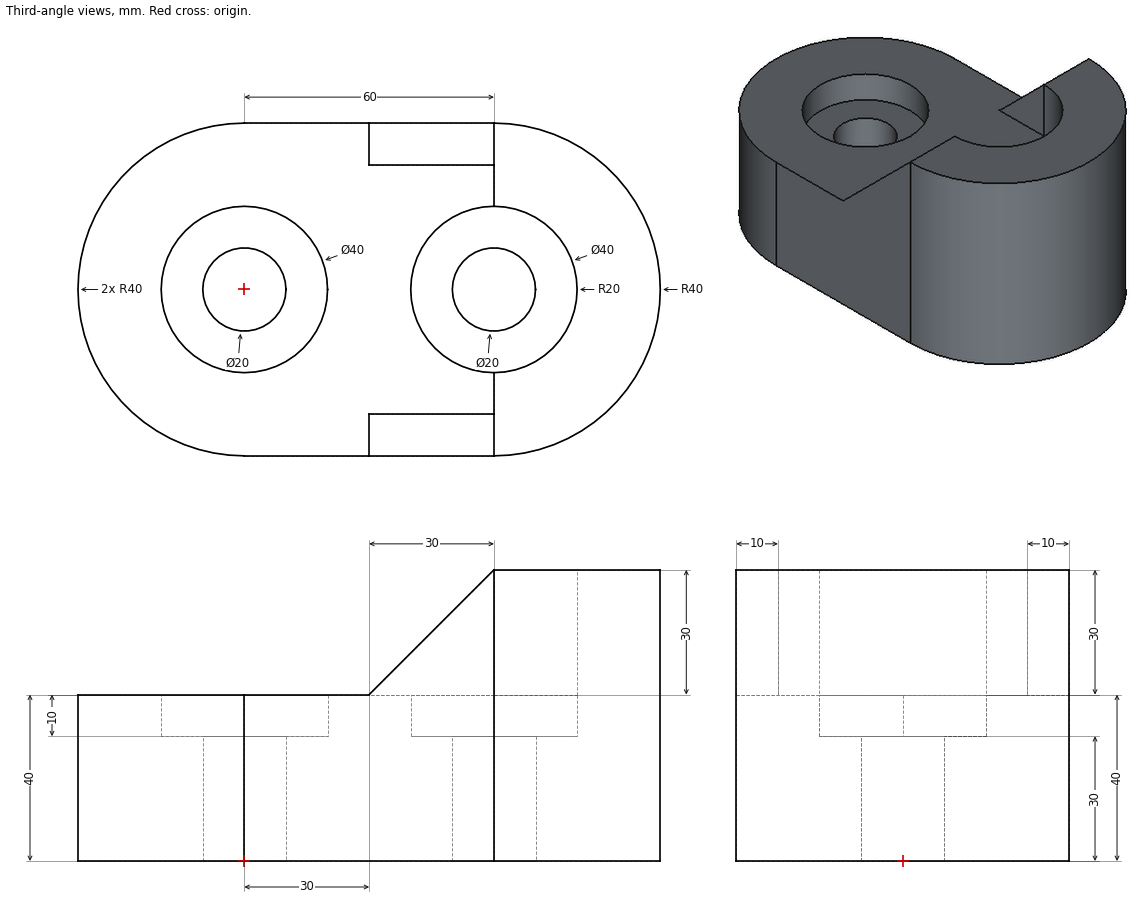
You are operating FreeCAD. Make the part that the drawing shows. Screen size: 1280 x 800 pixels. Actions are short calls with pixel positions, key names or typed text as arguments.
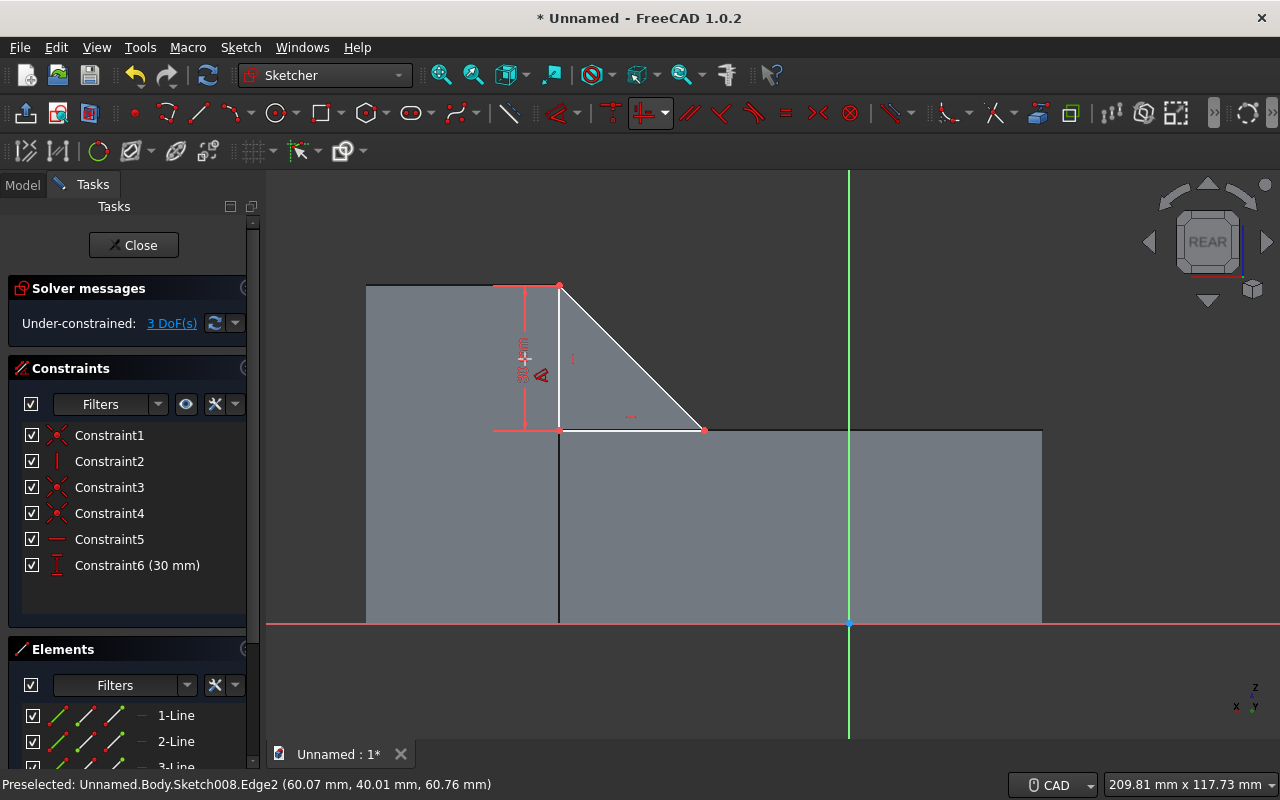
click(603, 431)
click(631, 397)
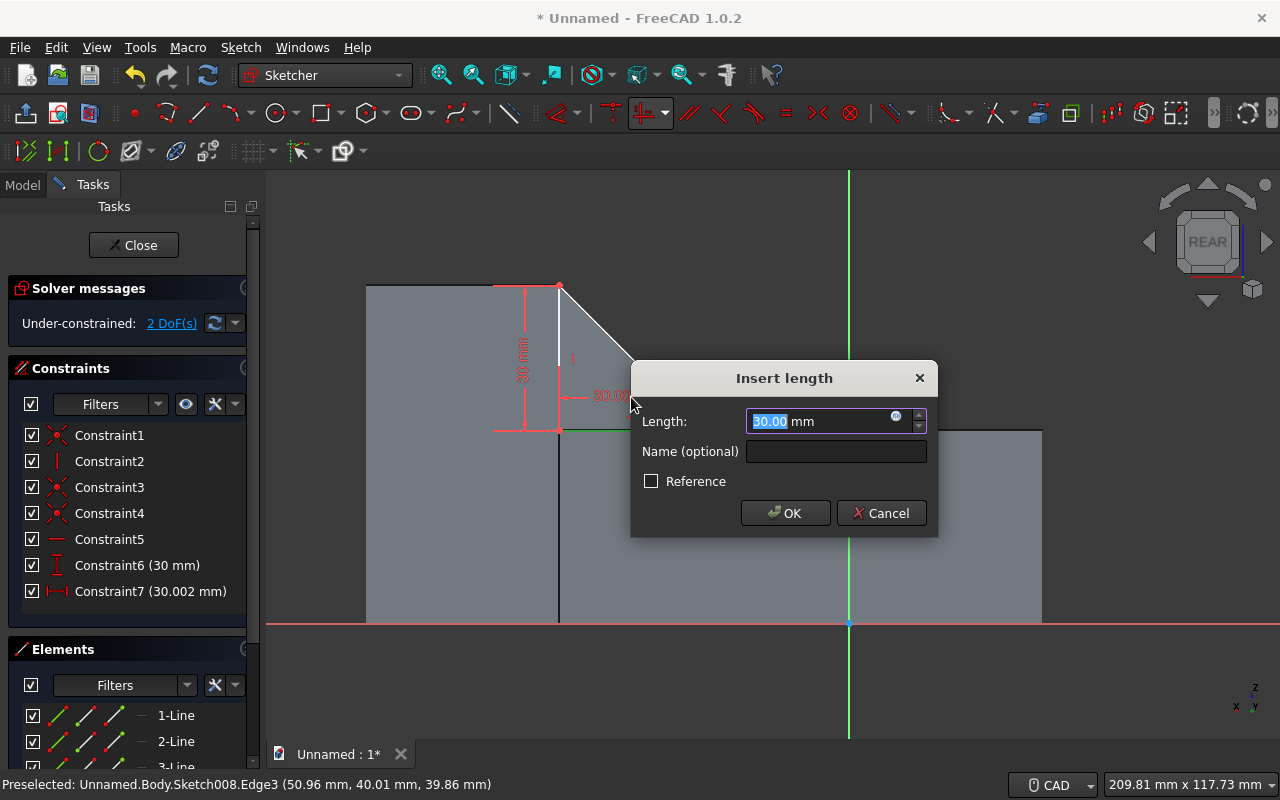
text(30)
key(Return)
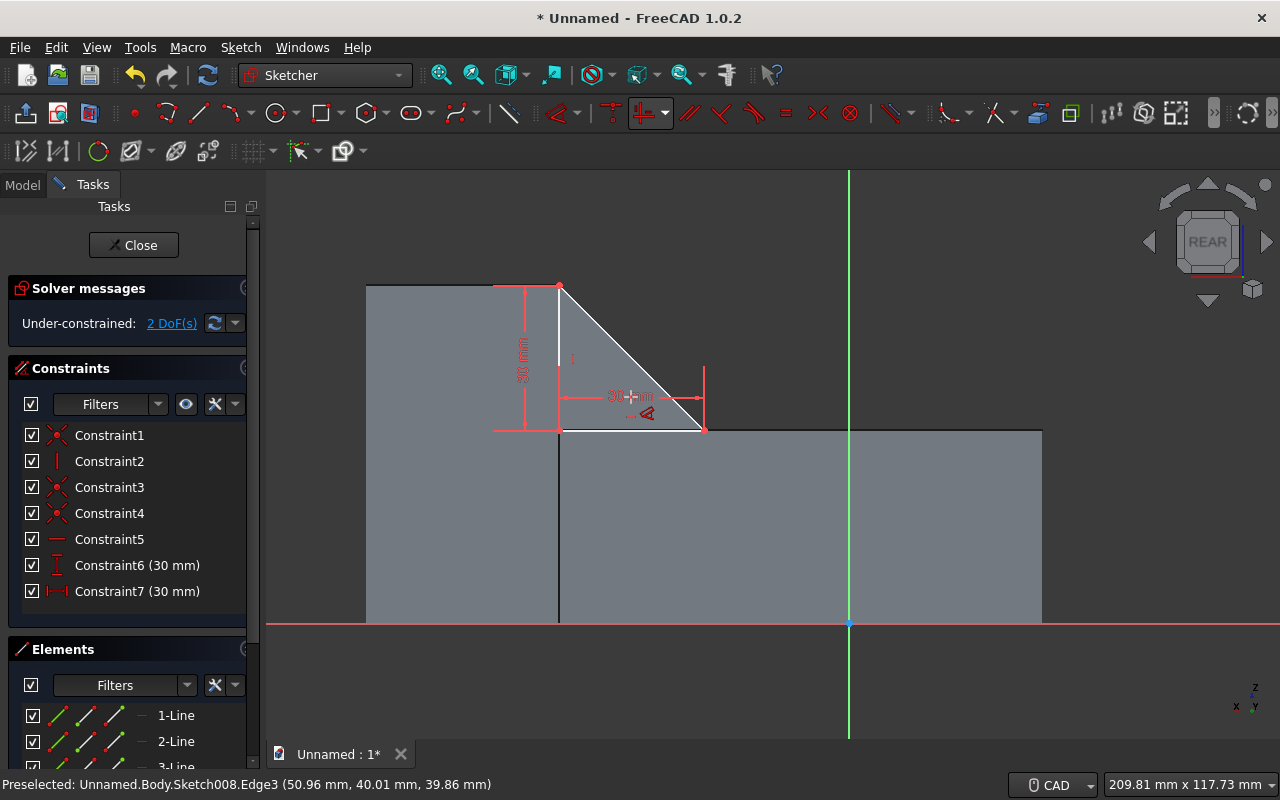
click(704, 431)
click(777, 658)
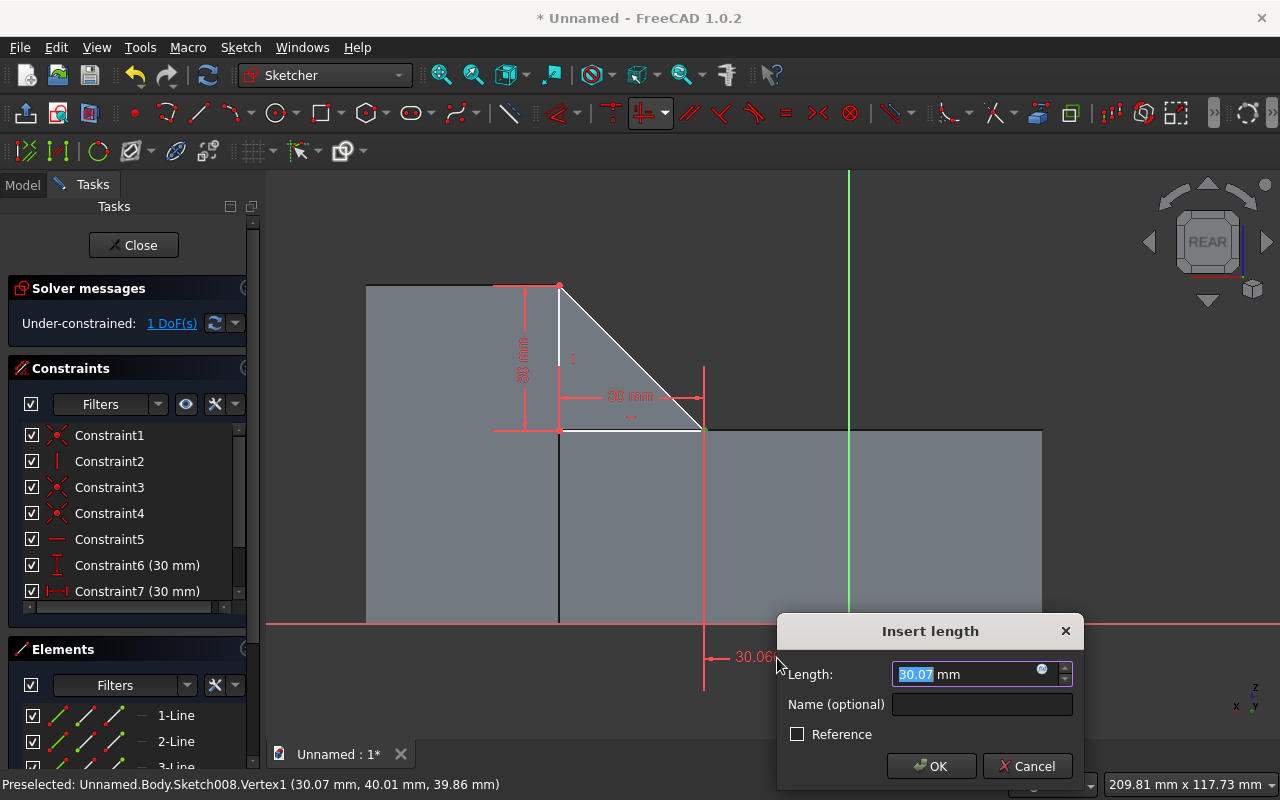
text(30)
key(Return)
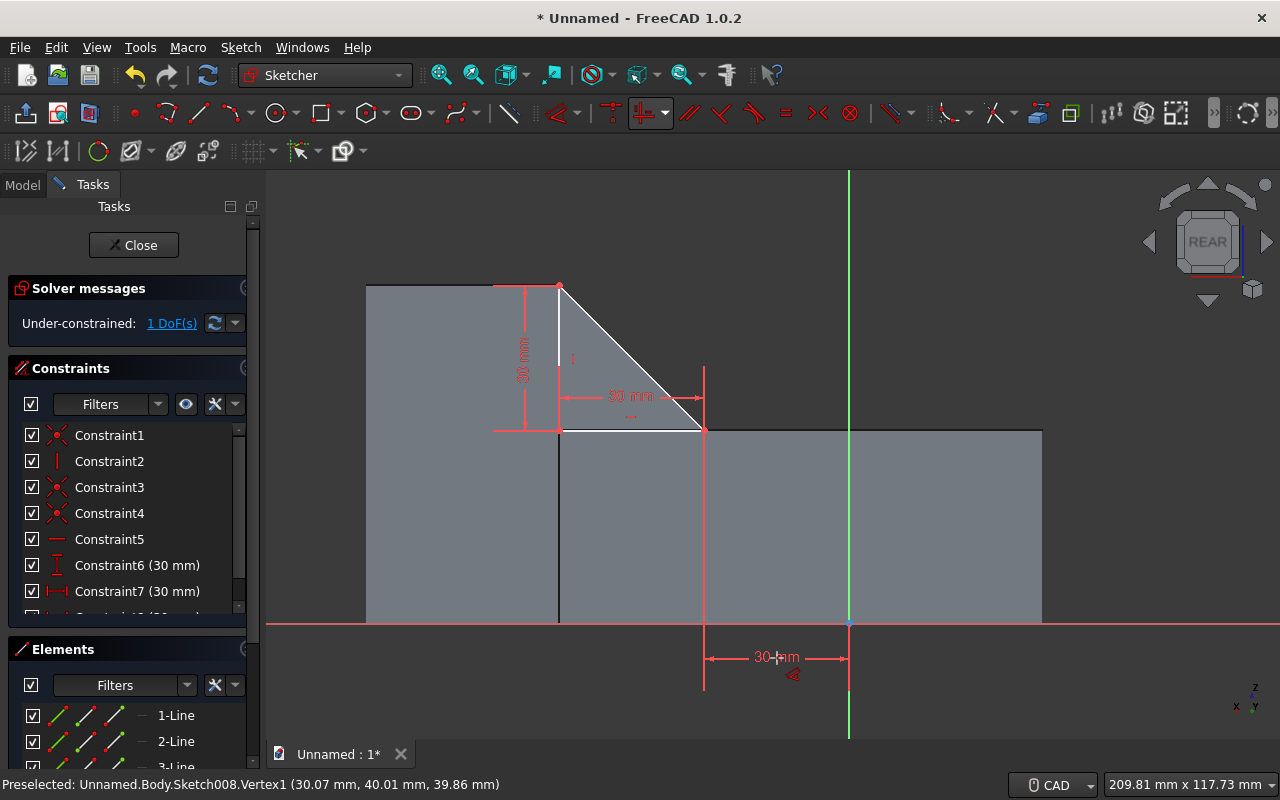
click(704, 431)
click(883, 527)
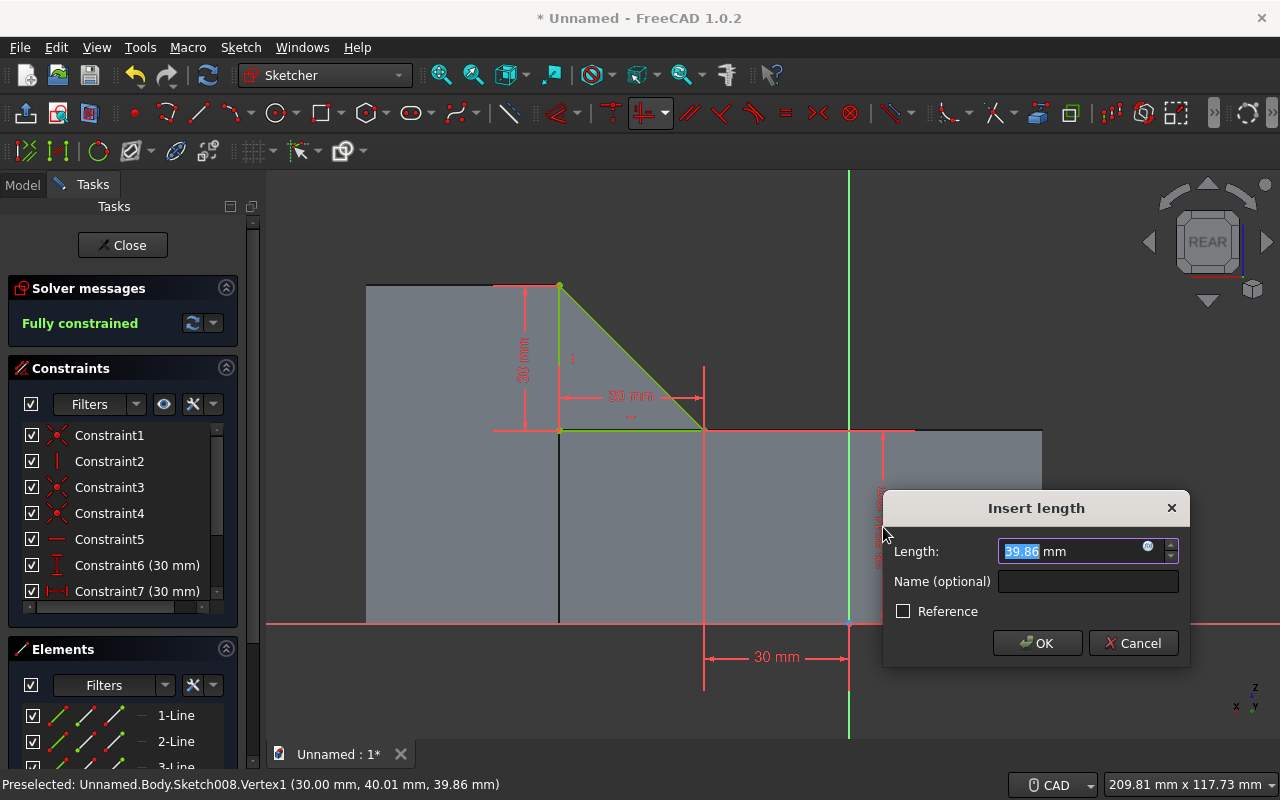
text(40)
key(Return)
key(Escape)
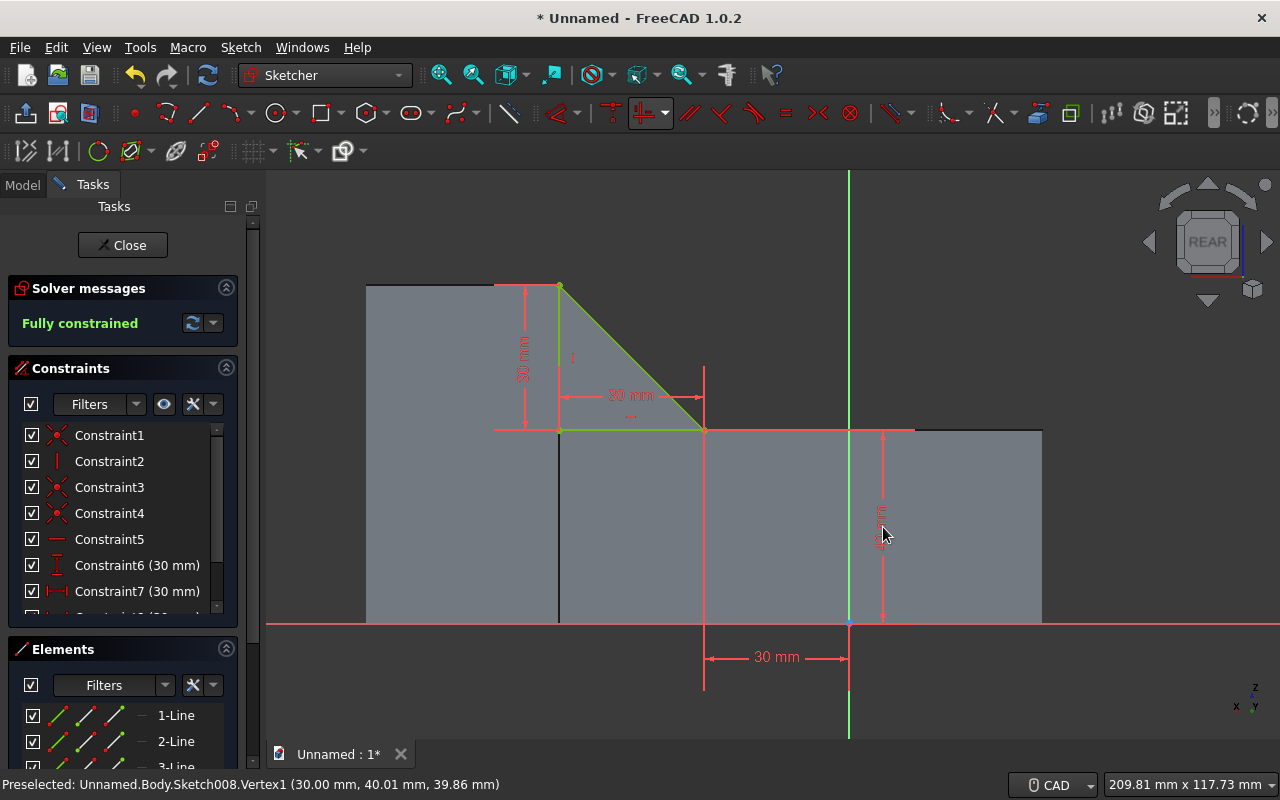
click(123, 245)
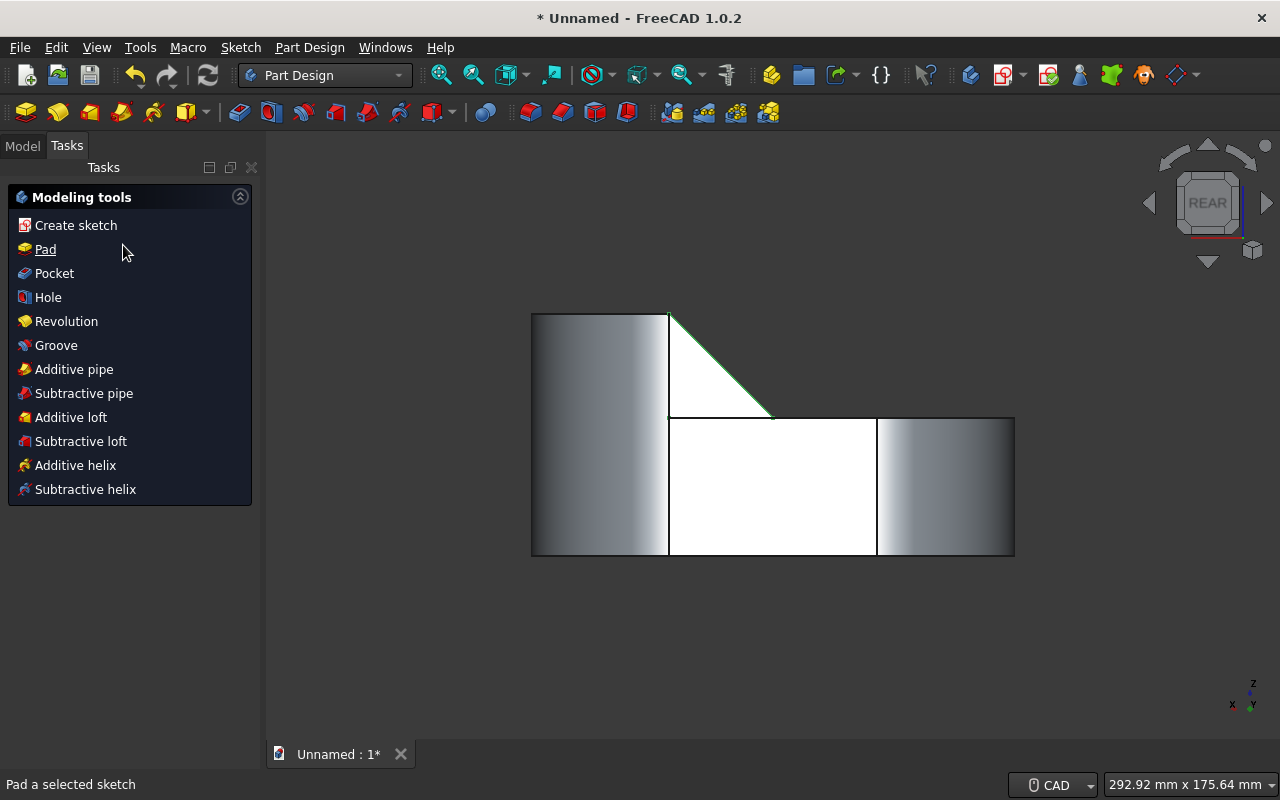
click(26, 112)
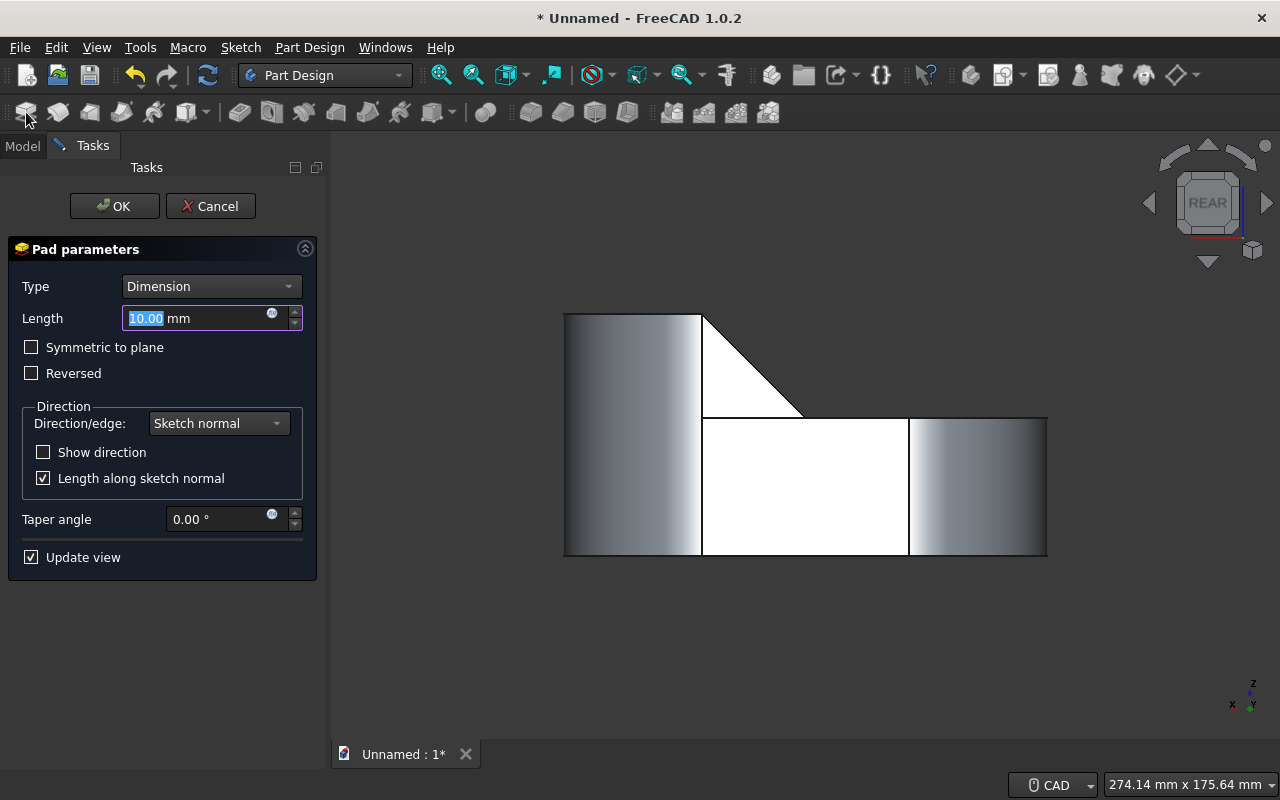
text(10)
key(Tab)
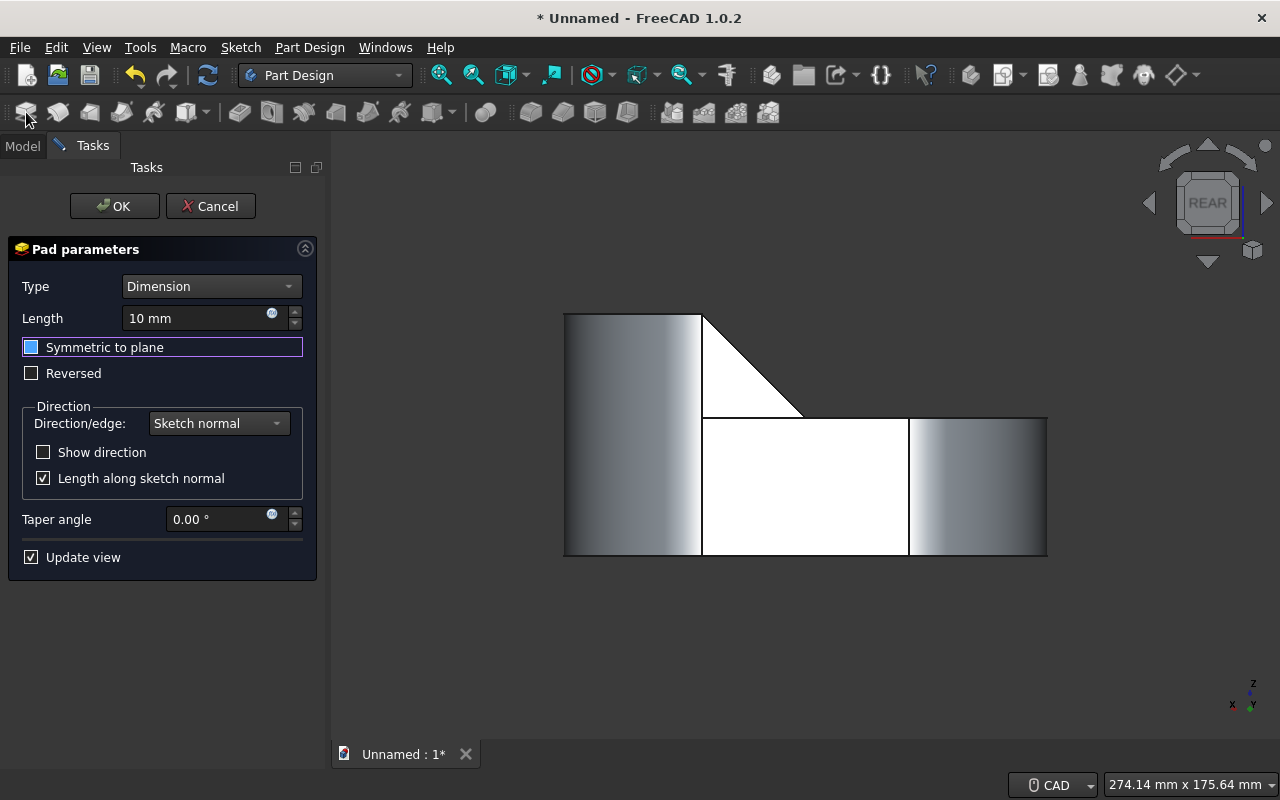
click(30, 373)